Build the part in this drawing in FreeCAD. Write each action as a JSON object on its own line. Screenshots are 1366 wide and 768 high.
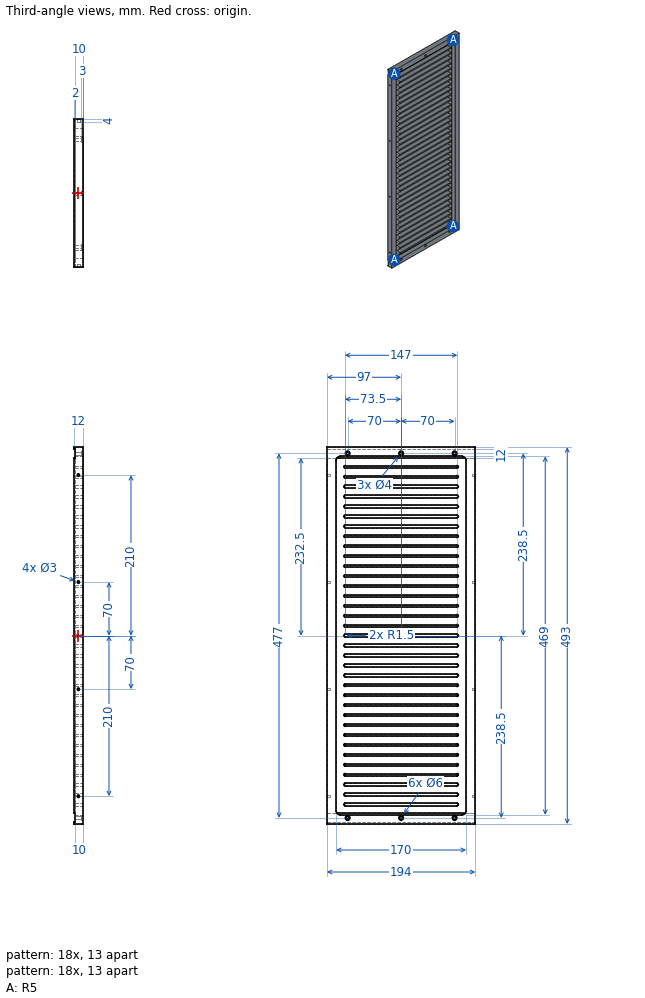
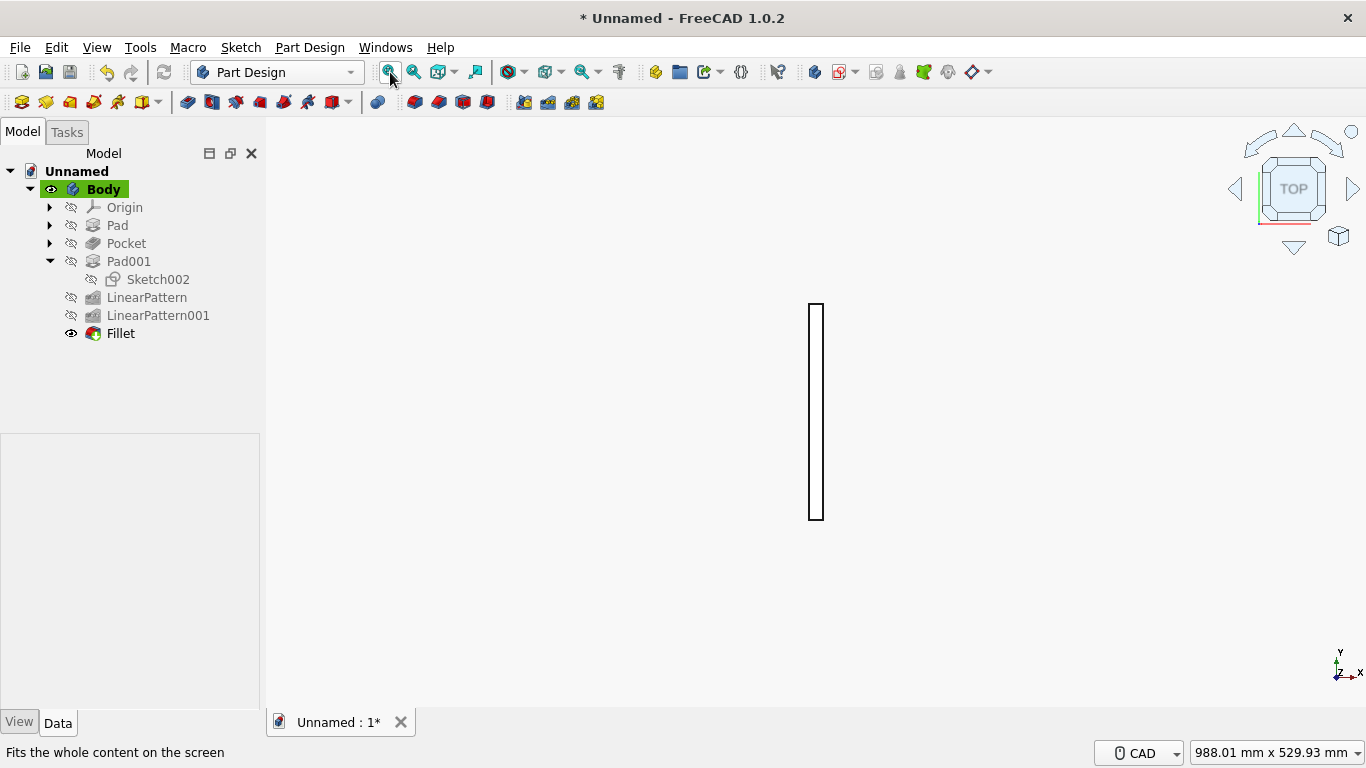
{"action": "left_click", "coordinate": [390, 72]}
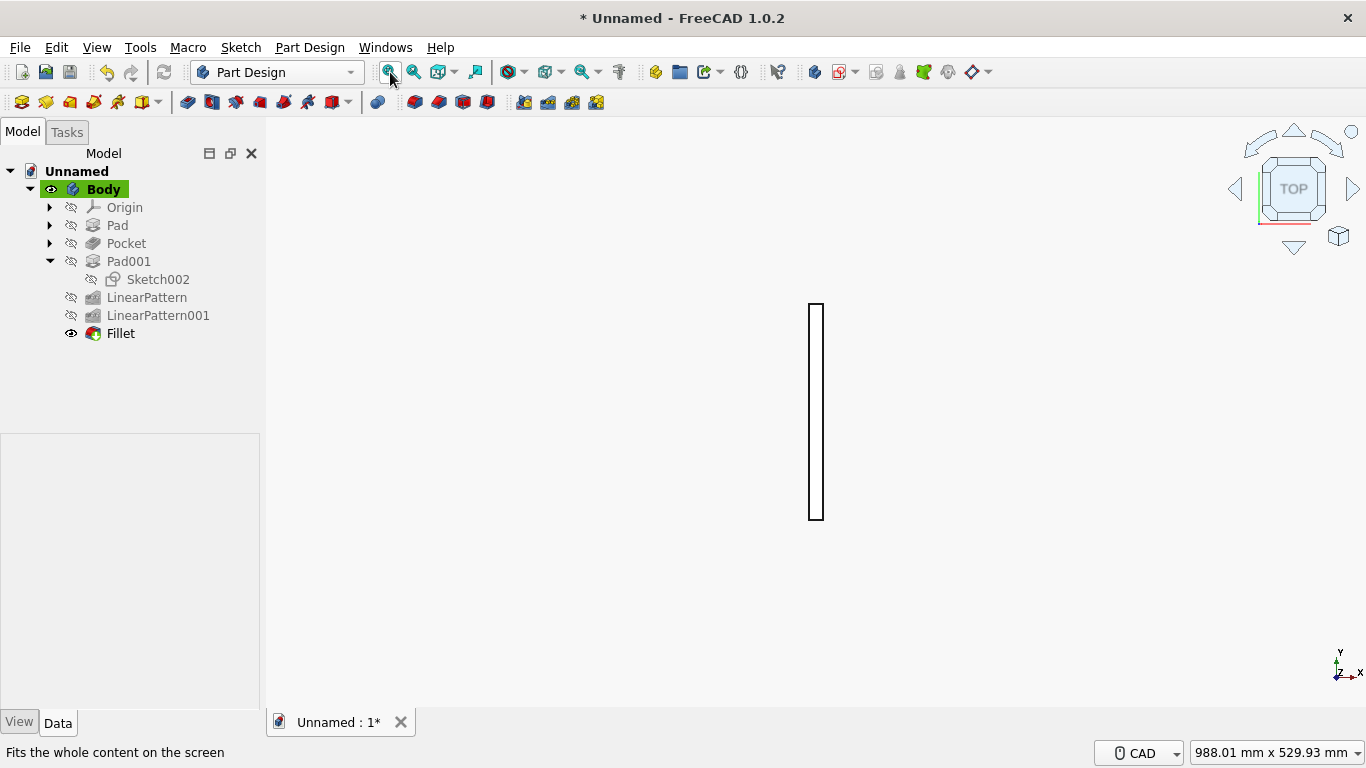
{"action": "left_click", "coordinate": [50, 207]}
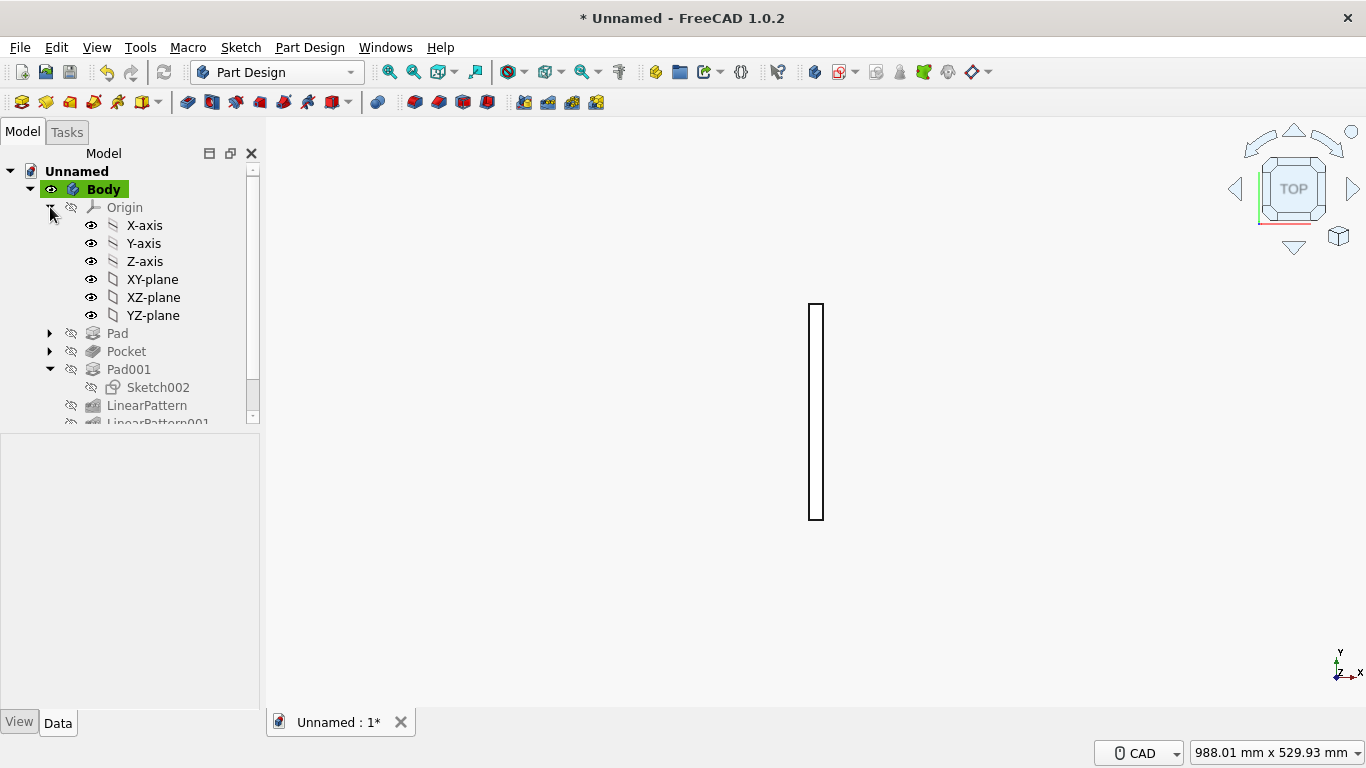
{"action": "left_click", "coordinate": [136, 315]}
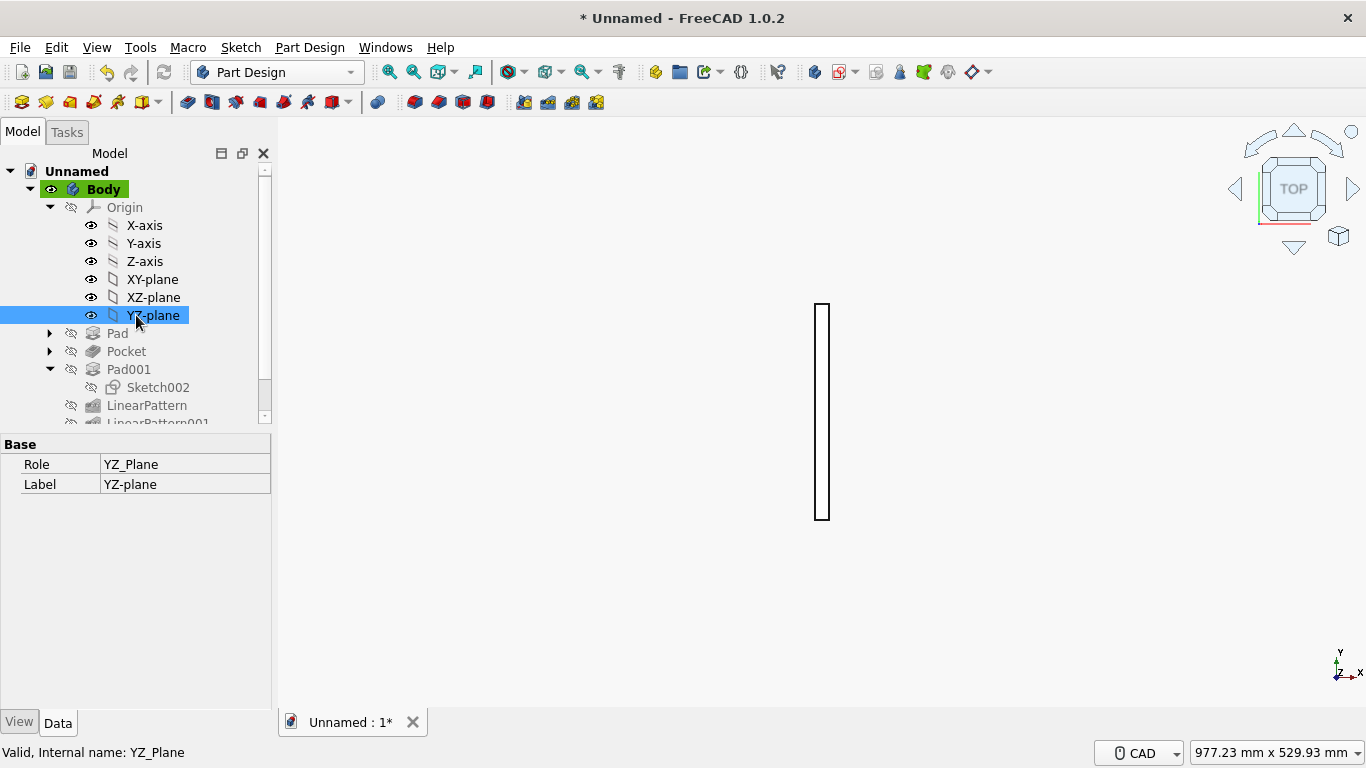
{"action": "left_click", "coordinate": [972, 72]}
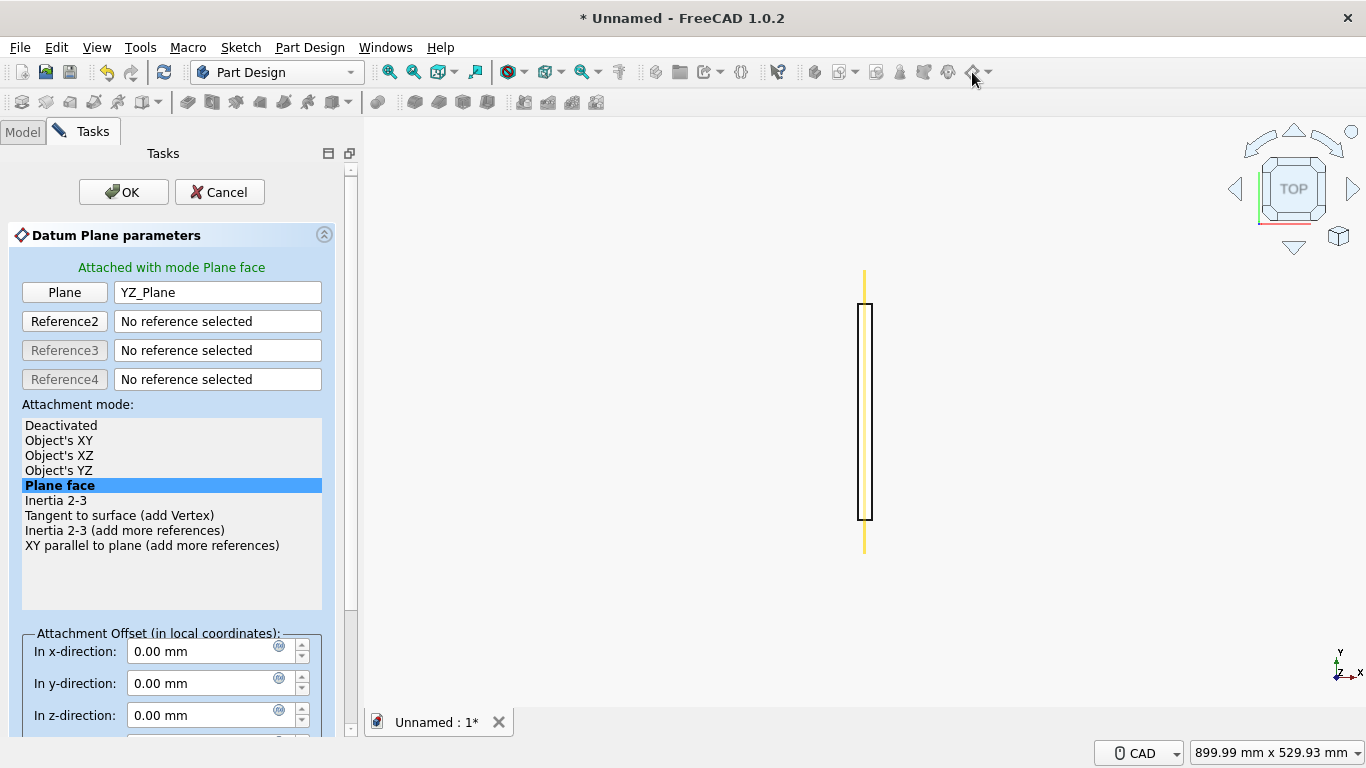
{"action": "triple_click", "coordinate": [210, 715]}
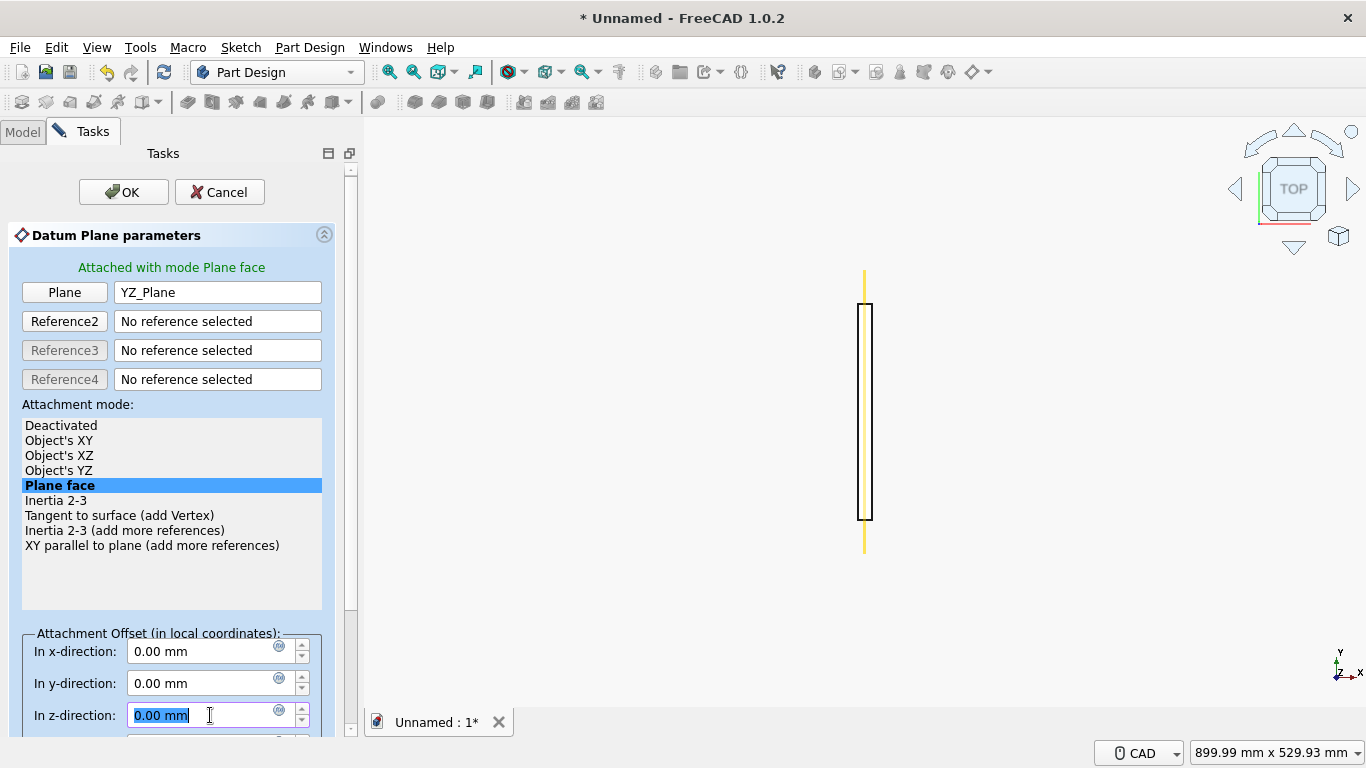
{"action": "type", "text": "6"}
{"action": "key", "text": "Tab"}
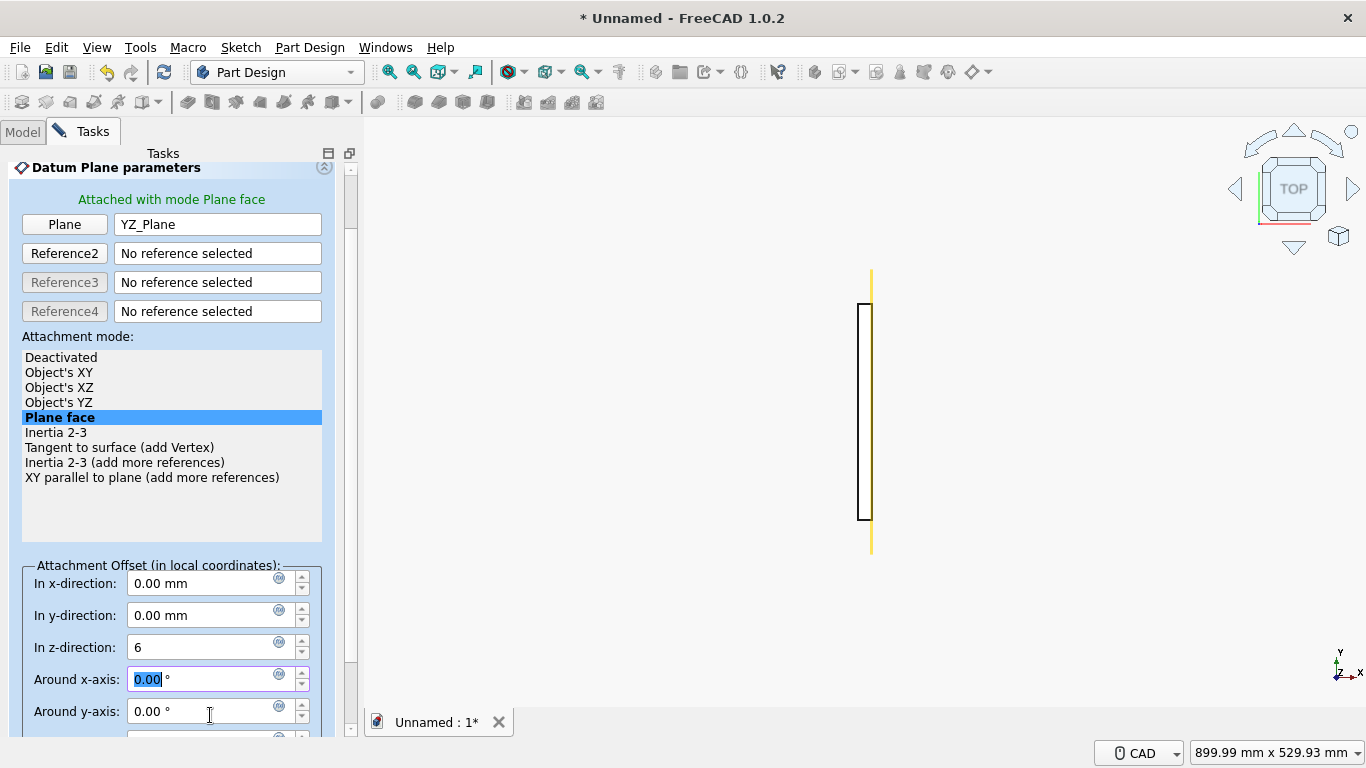
{"action": "scroll", "coordinate": [351, 450], "scroll_direction": "up", "scroll_amount": 2}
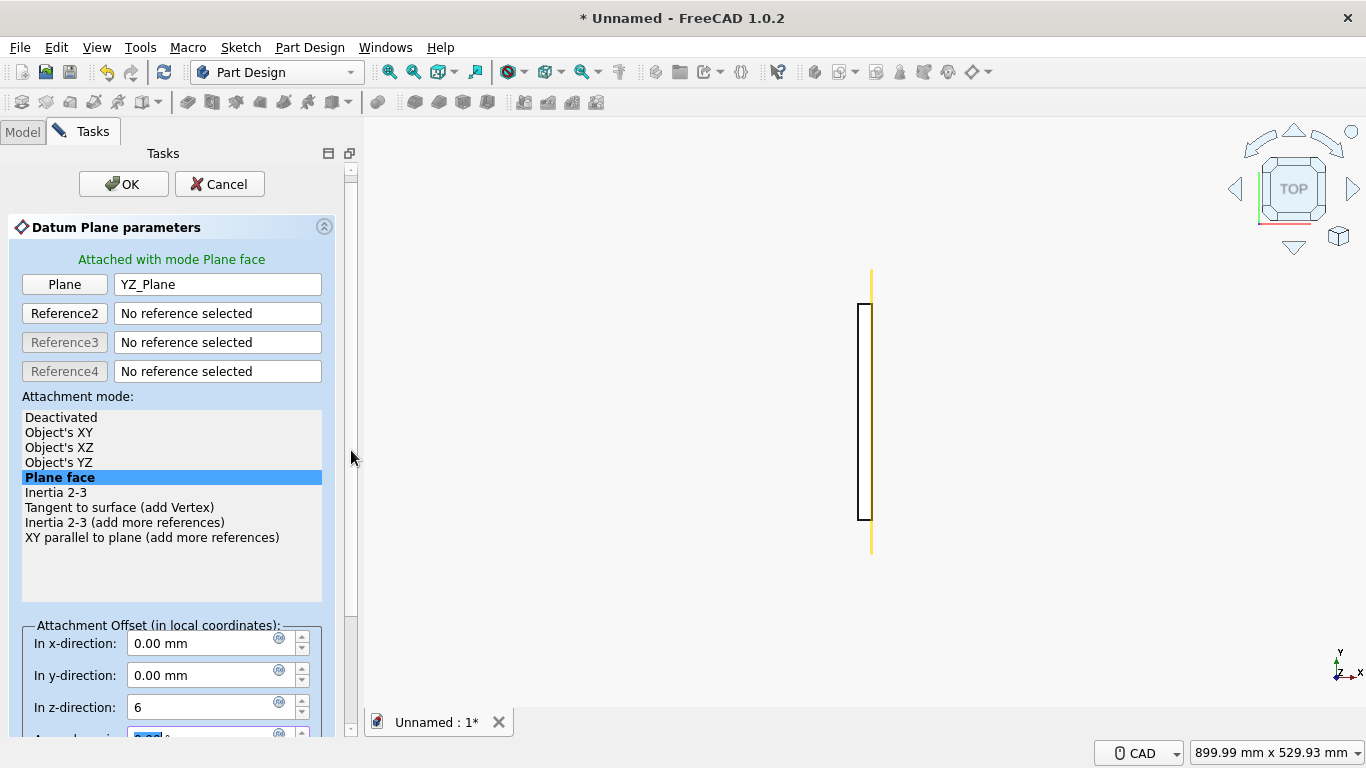
{"action": "left_click", "coordinate": [124, 192]}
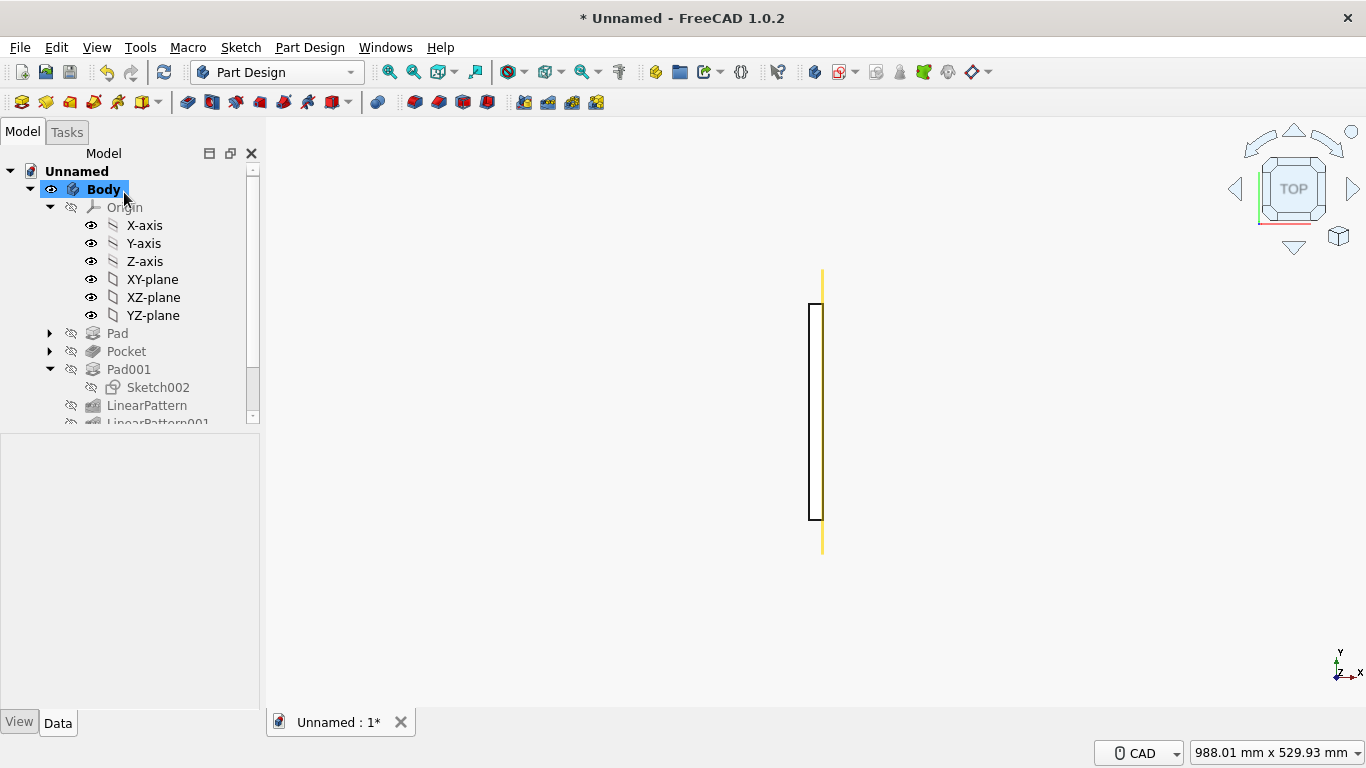
{"action": "scroll", "coordinate": [100, 293], "scroll_direction": "down", "scroll_amount": 3}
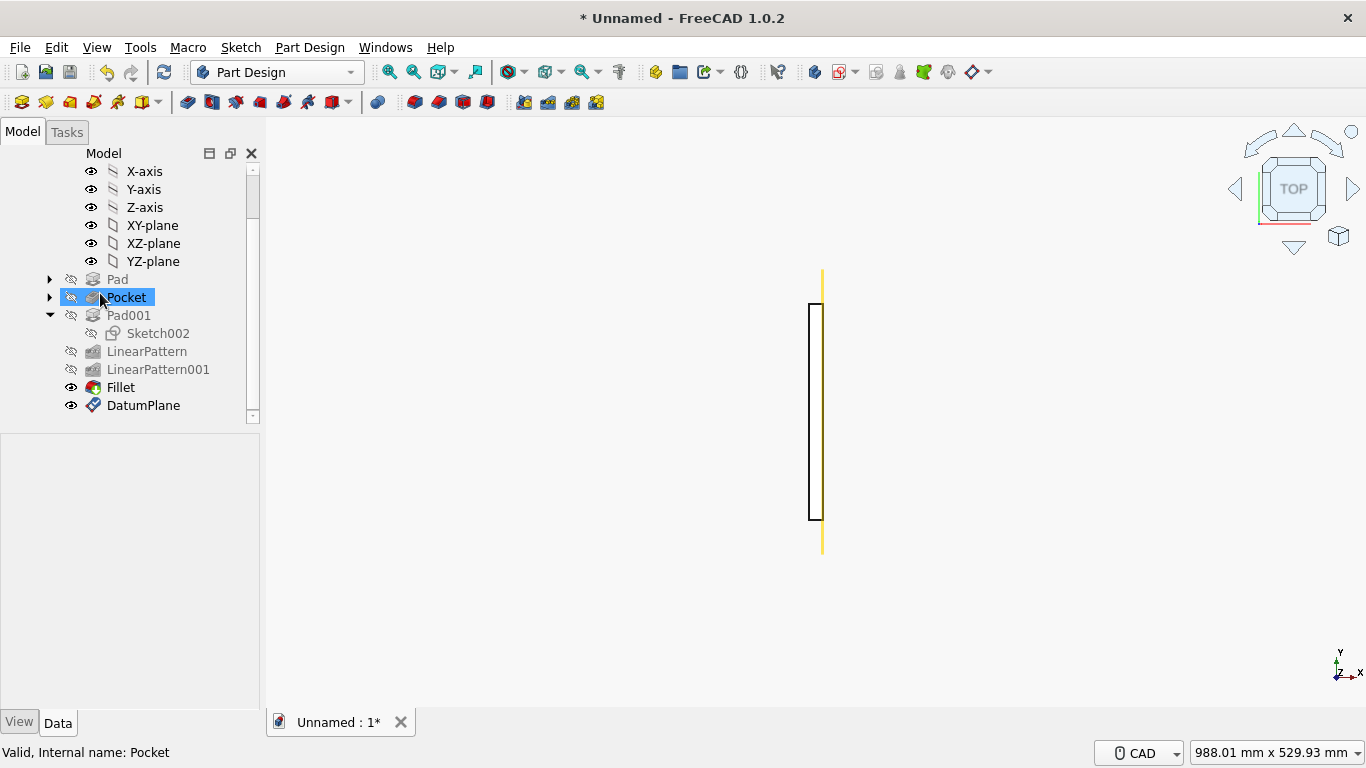
{"action": "left_click", "coordinate": [116, 405]}